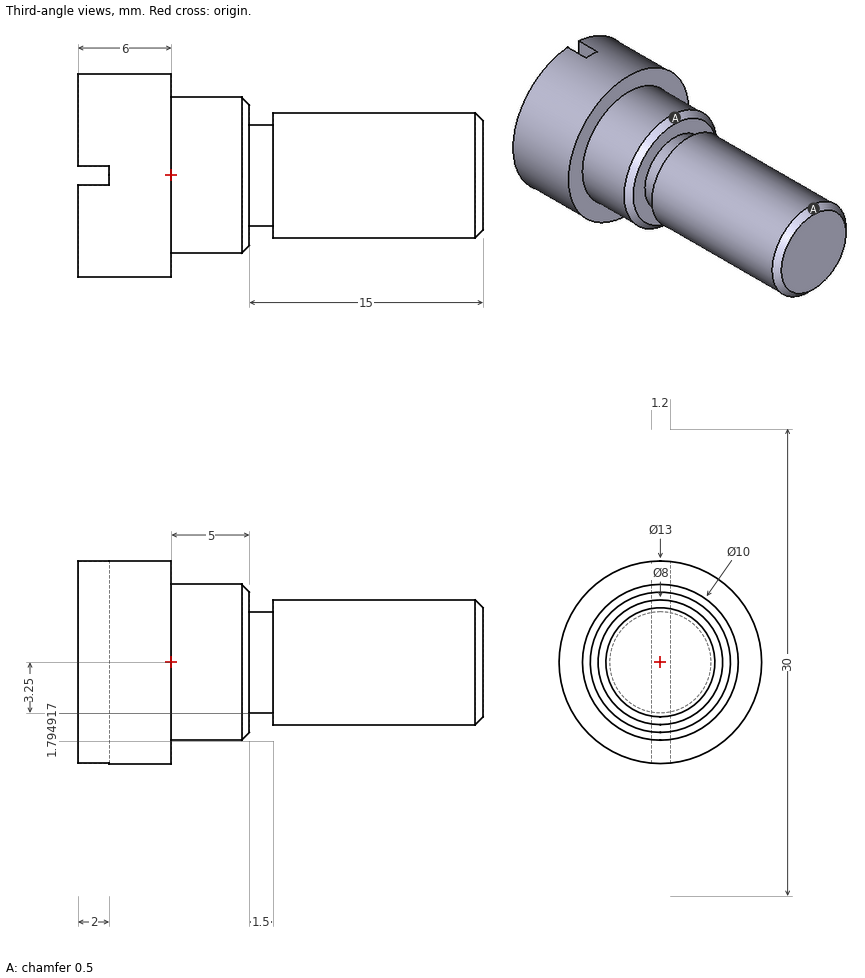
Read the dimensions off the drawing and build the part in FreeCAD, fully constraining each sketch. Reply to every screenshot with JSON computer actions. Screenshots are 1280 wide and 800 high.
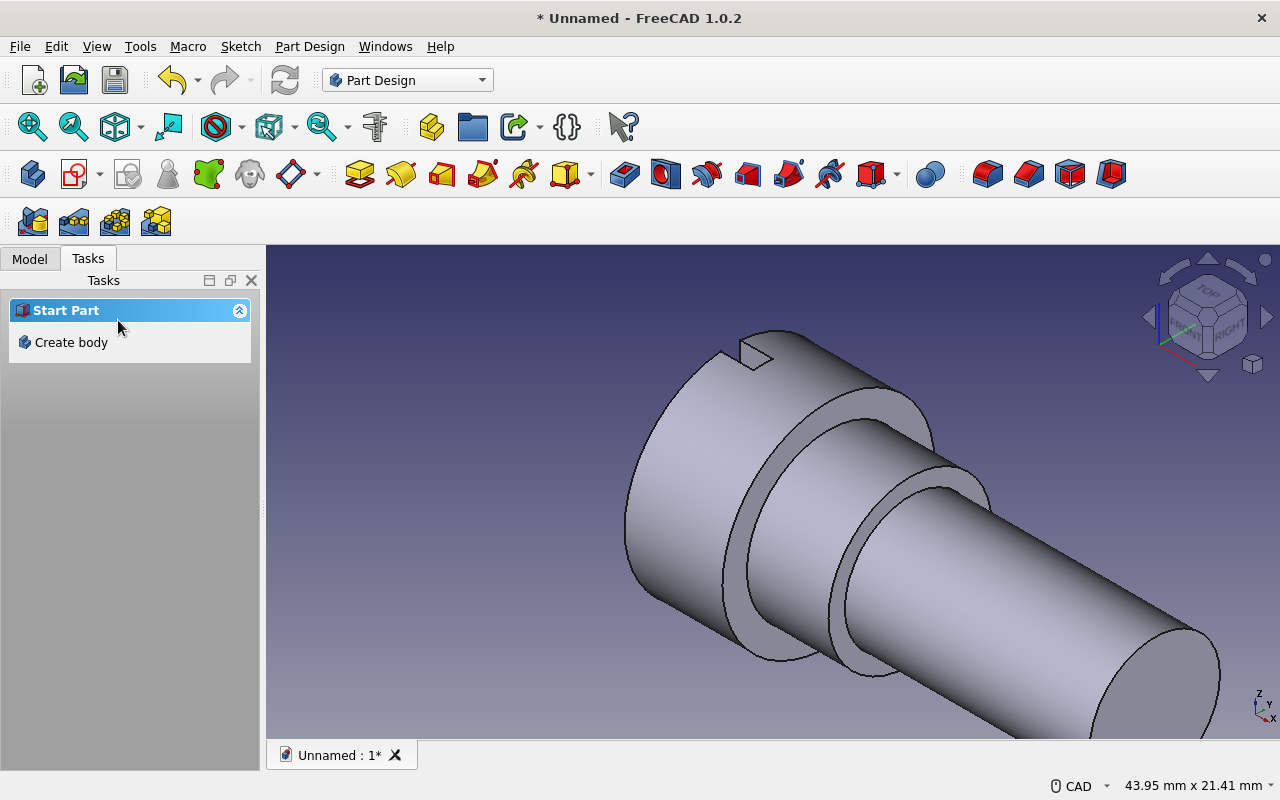
{"action": "key", "text": "v f"}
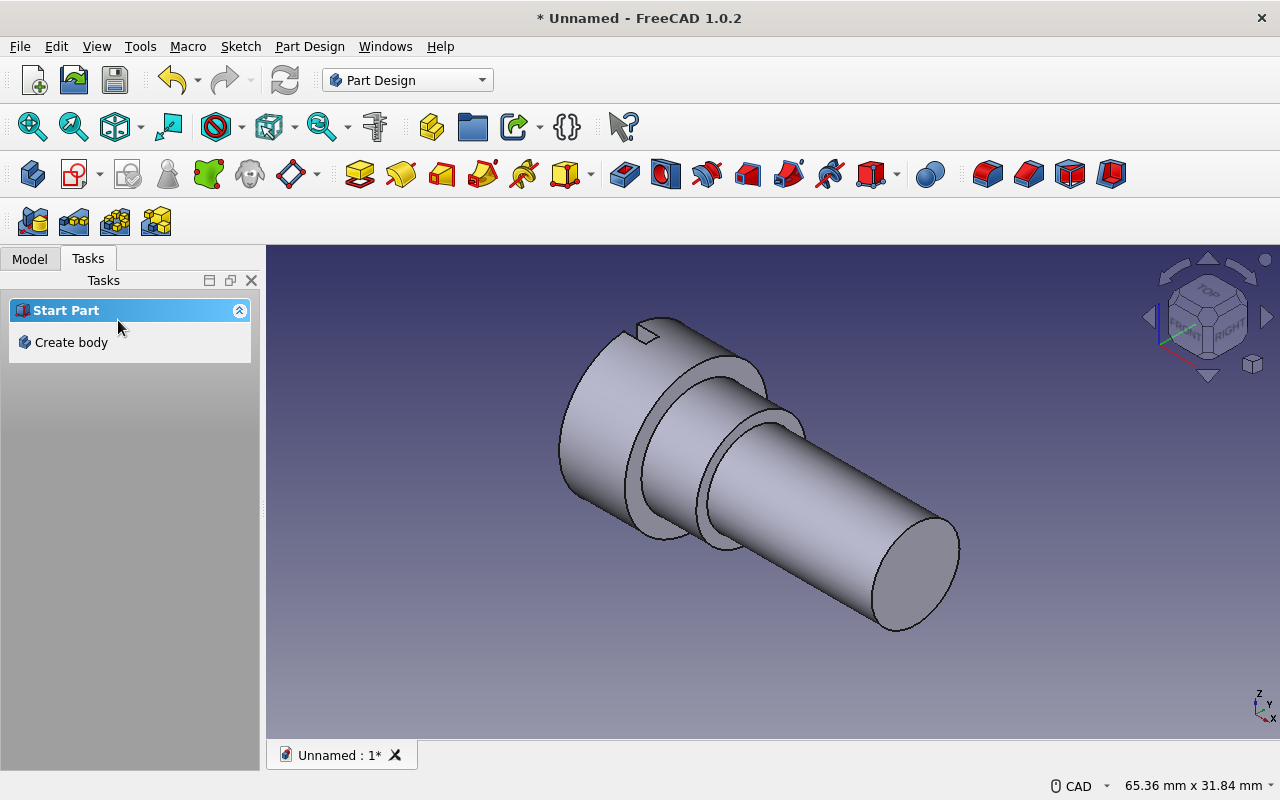
{"action": "left_click", "coordinate": [872, 599]}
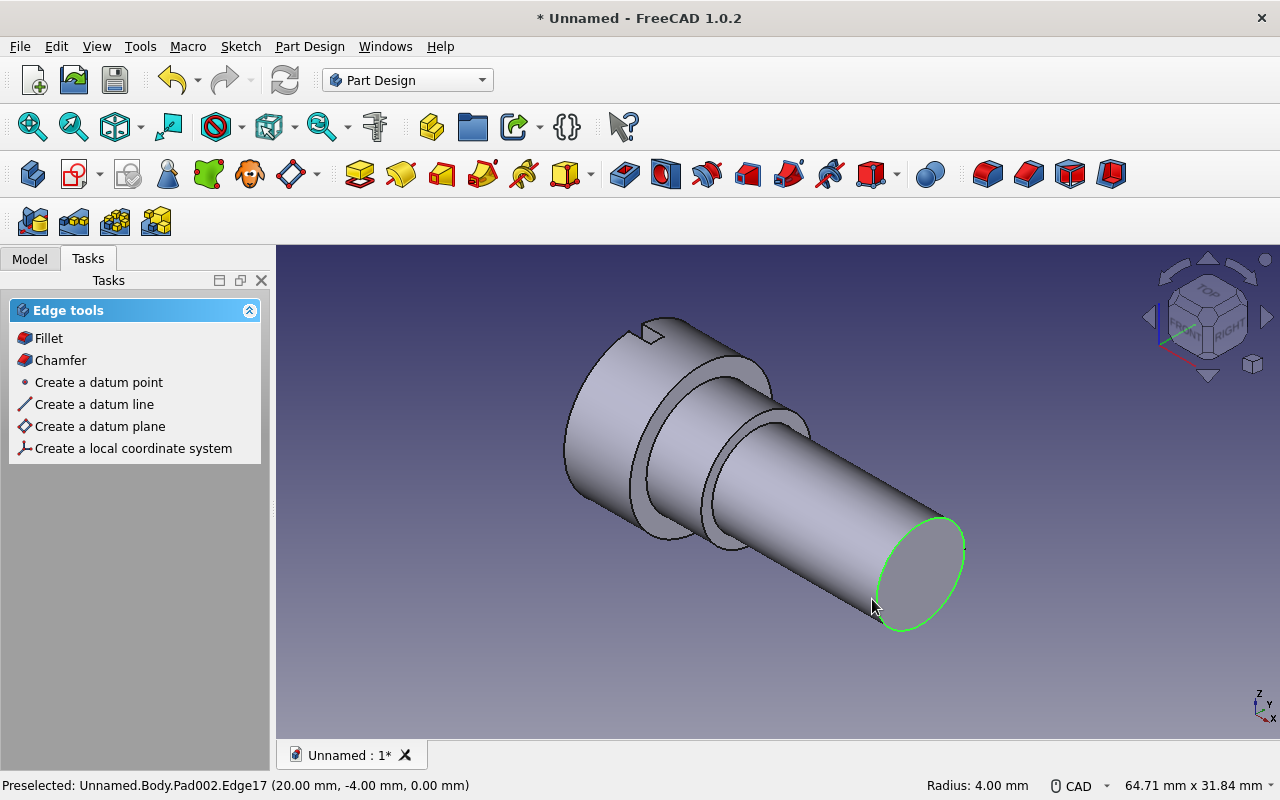
{"action": "left_click", "coordinate": [701, 510], "text": "ctrl"}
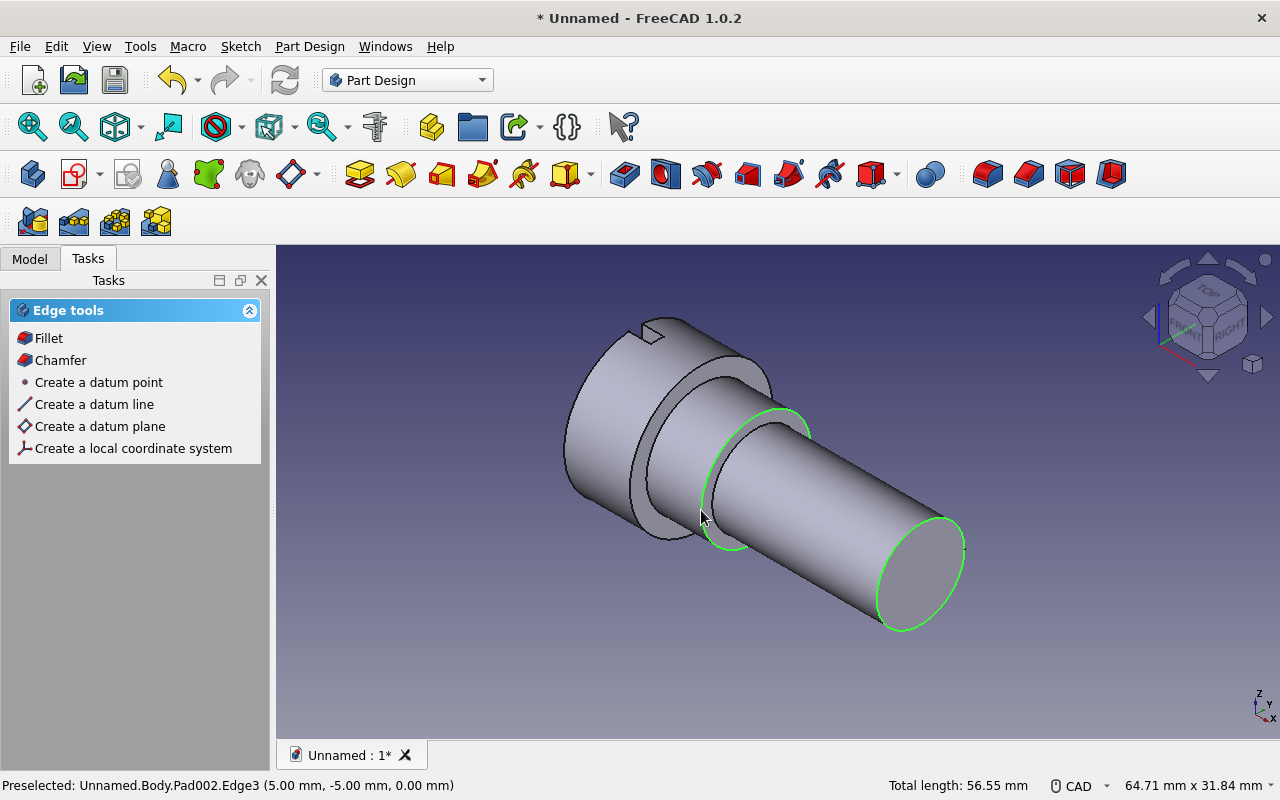
{"action": "left_click", "coordinate": [1029, 174]}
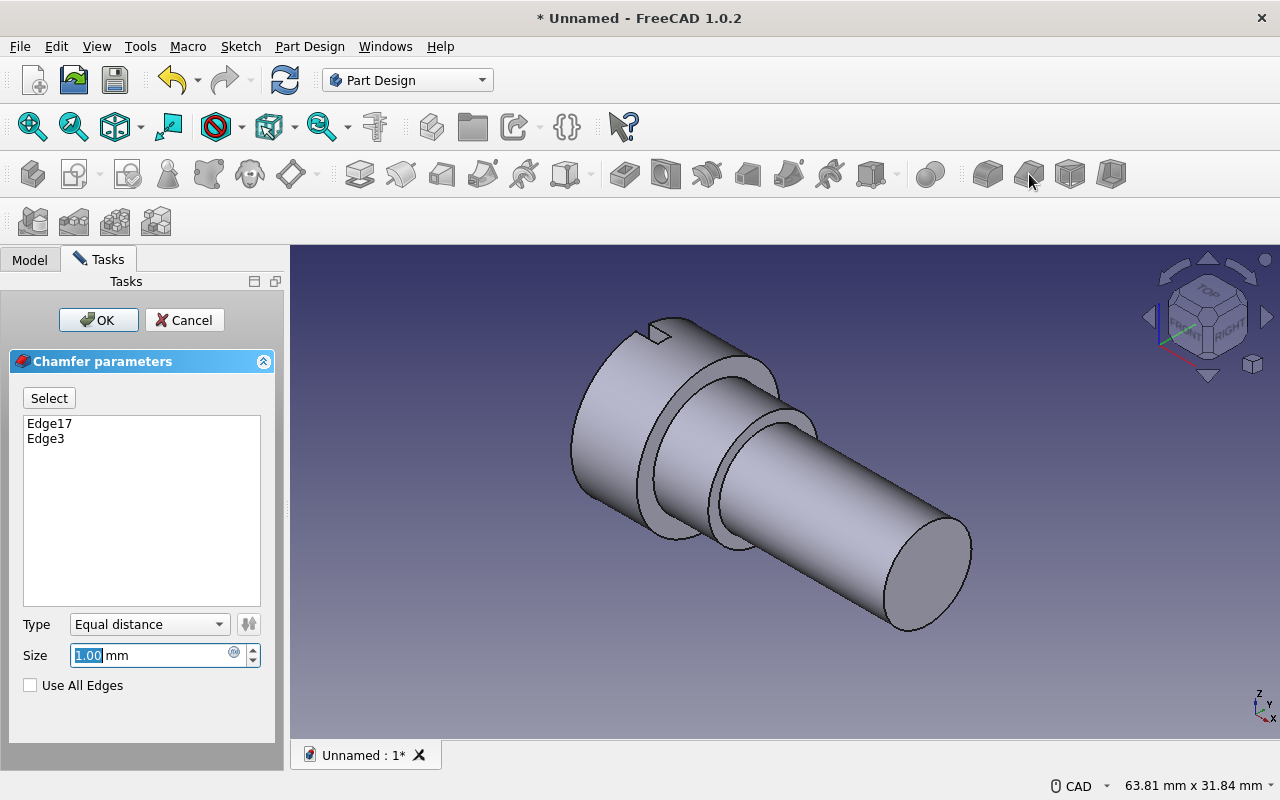
{"action": "type", "text": "0.5"}
{"action": "key", "text": "Tab"}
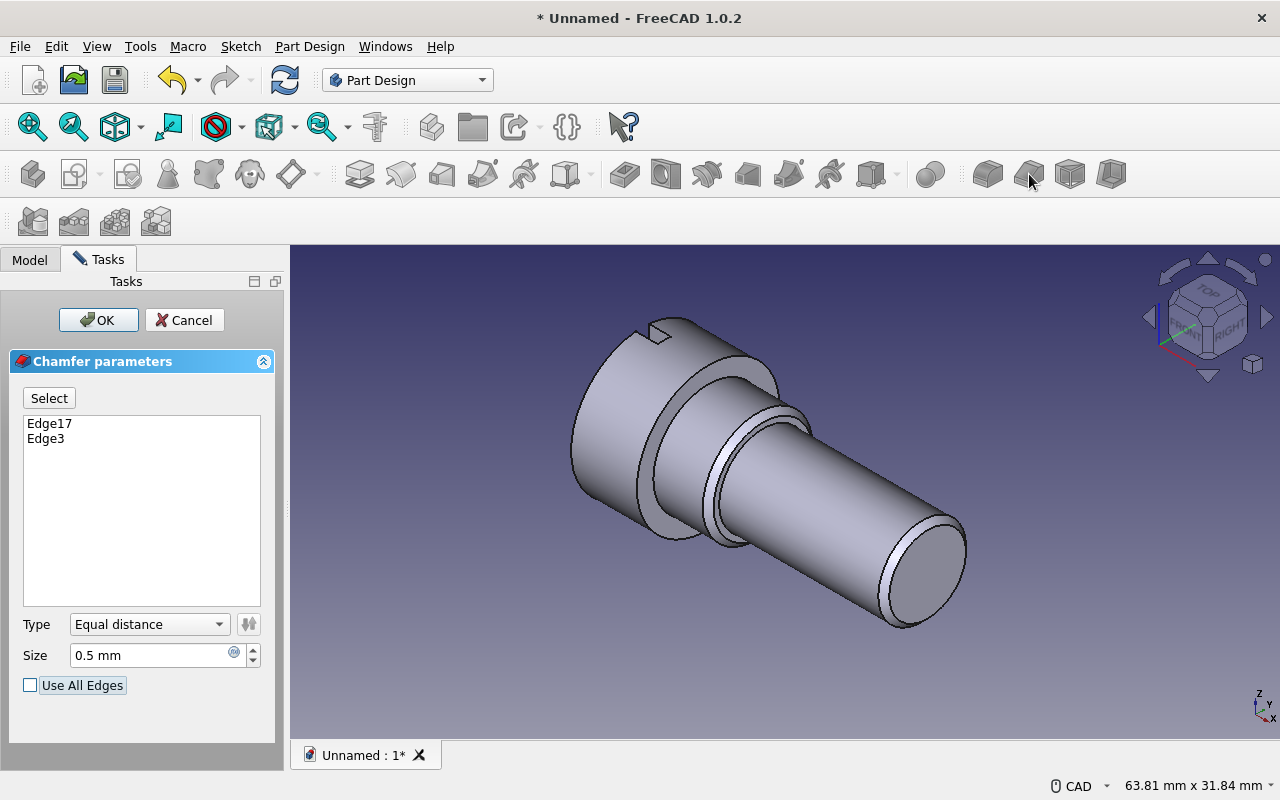
{"action": "left_click", "coordinate": [99, 320]}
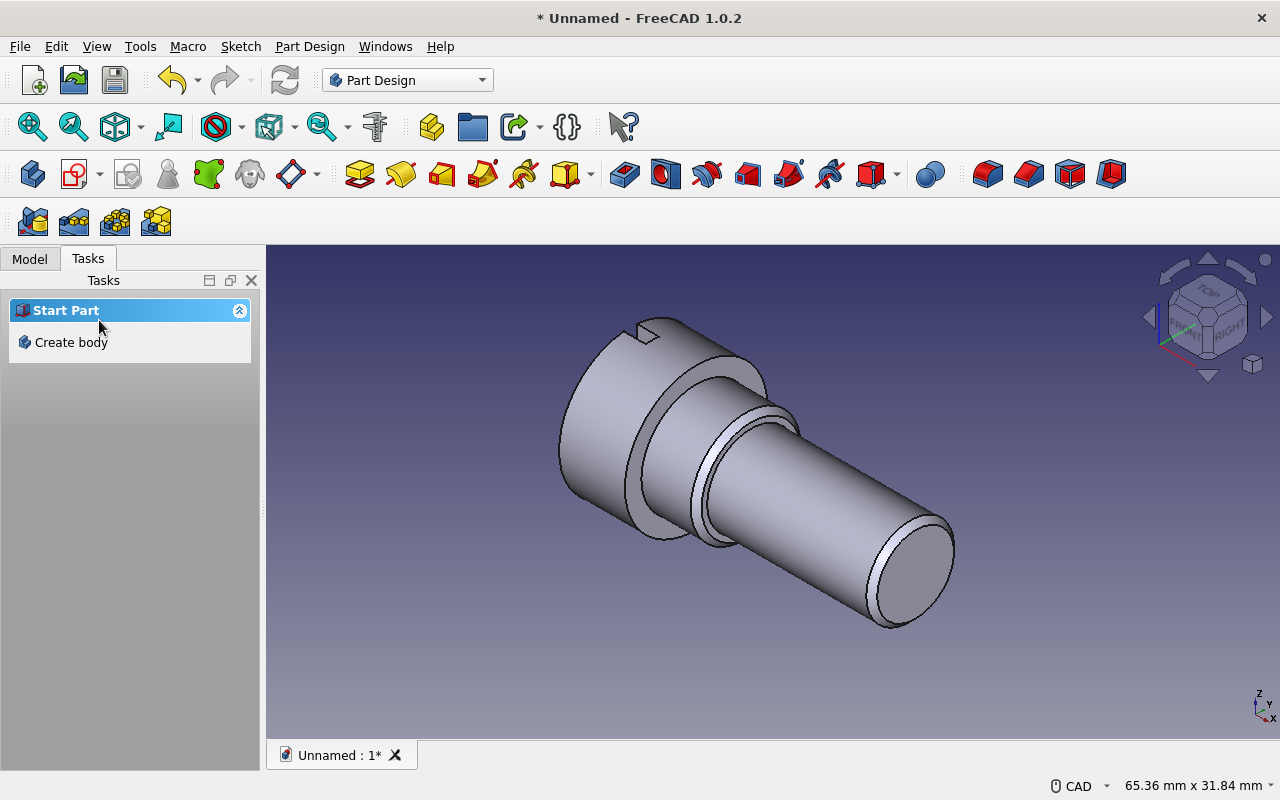
{"action": "left_click", "coordinate": [74, 174]}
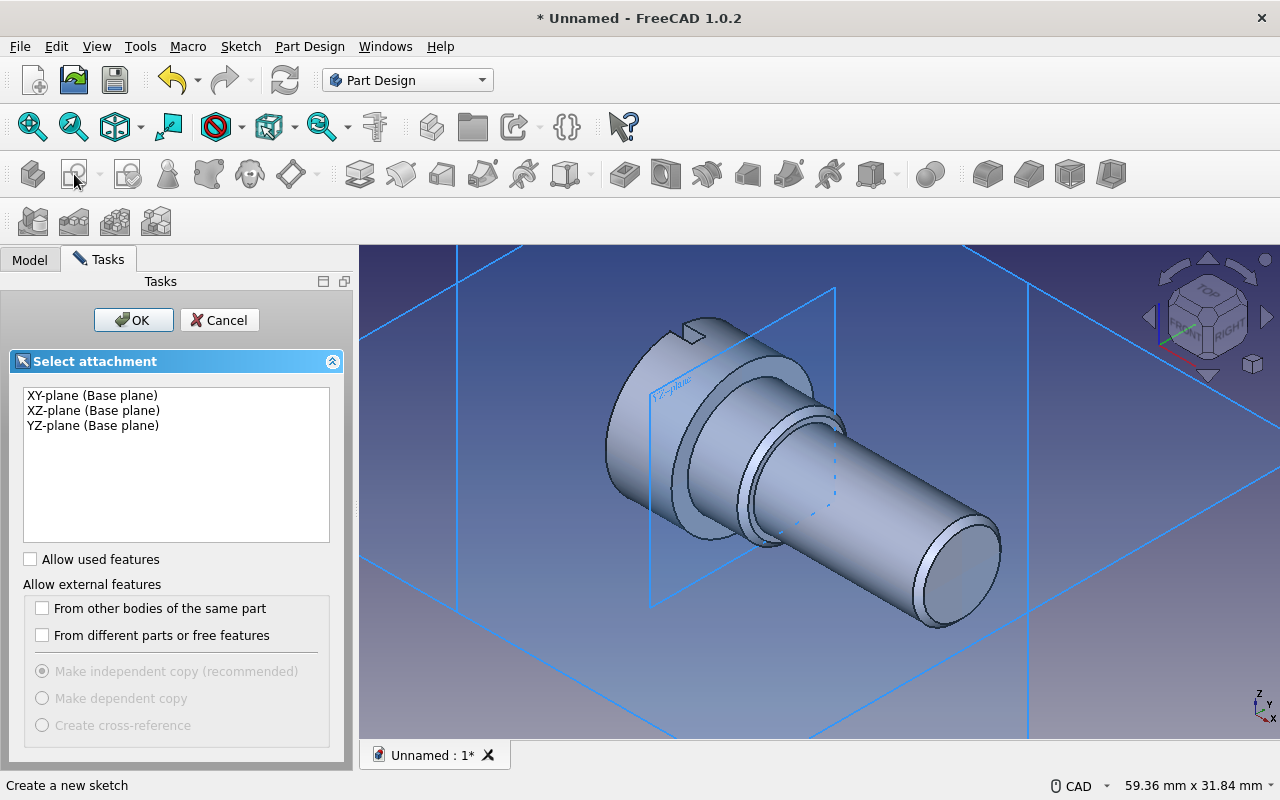
{"action": "left_click", "coordinate": [84, 410]}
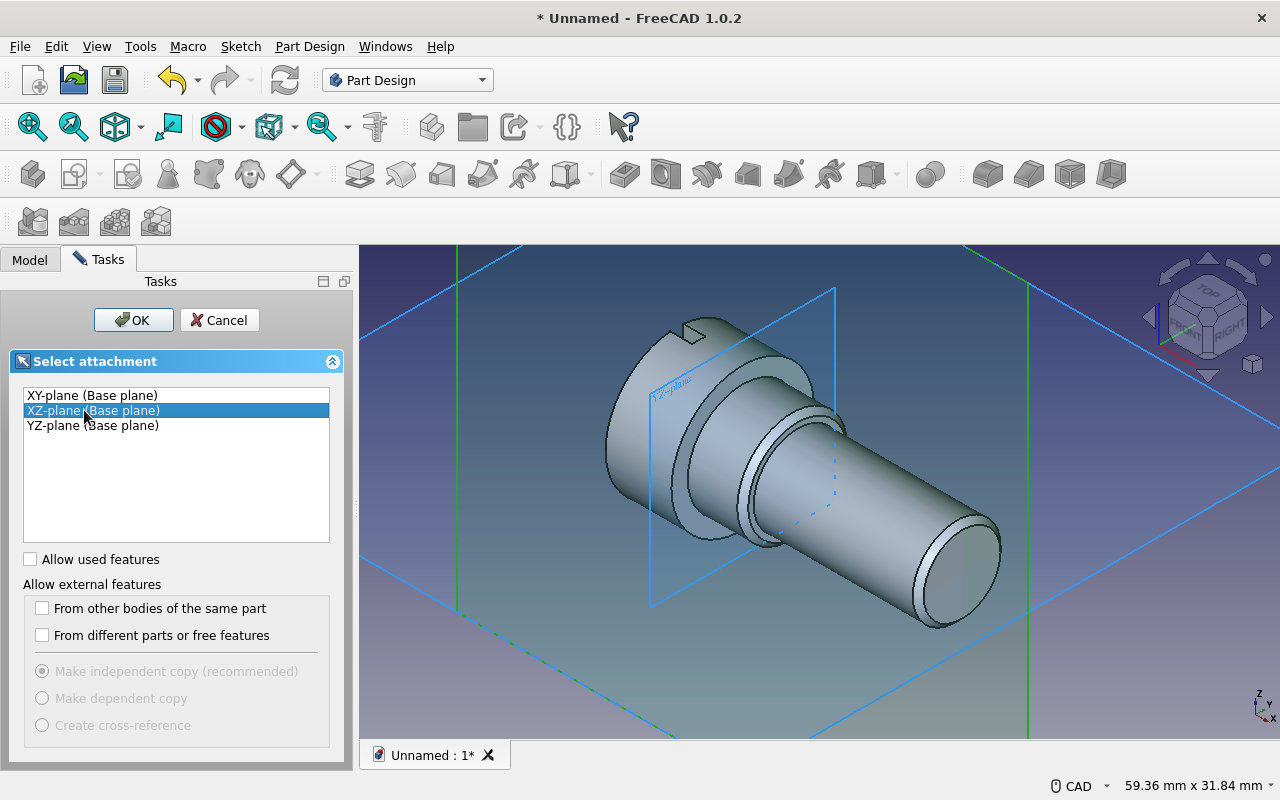
{"action": "left_click", "coordinate": [134, 320]}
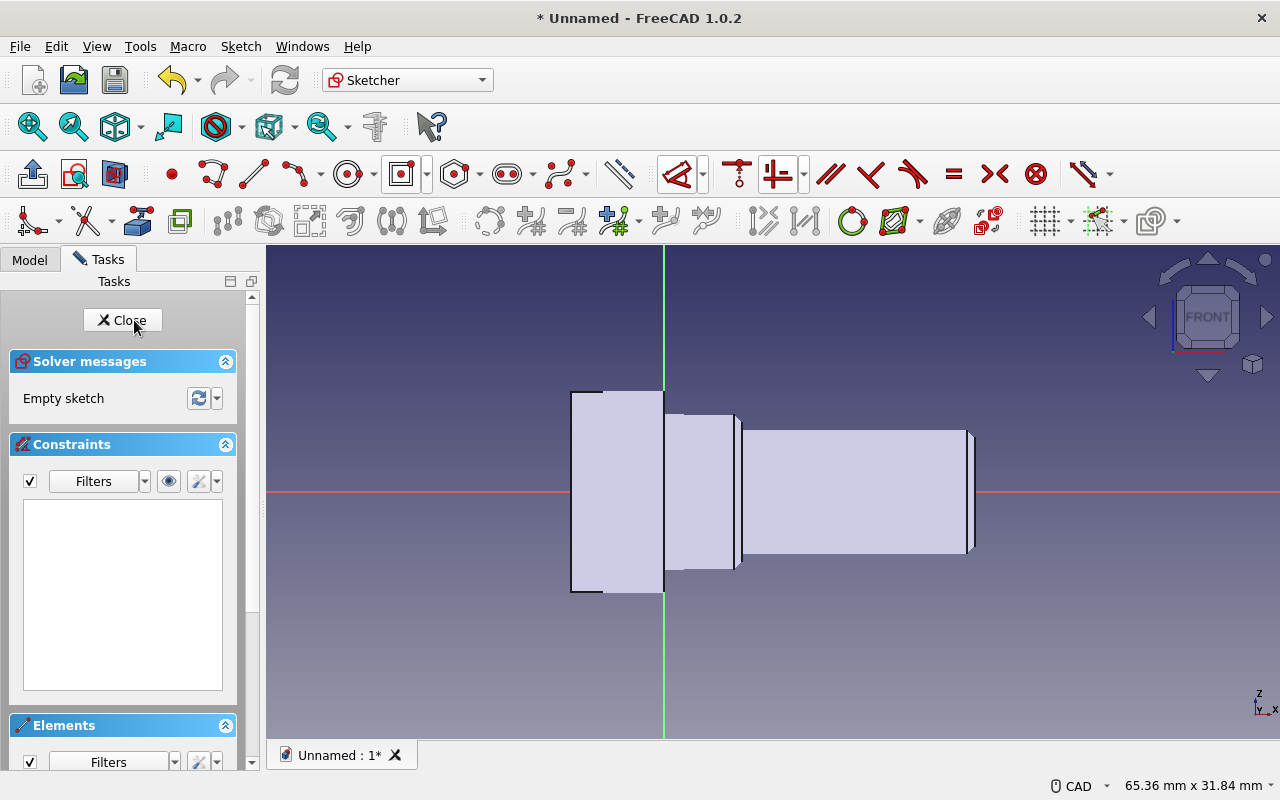
{"action": "left_click", "coordinate": [115, 174]}